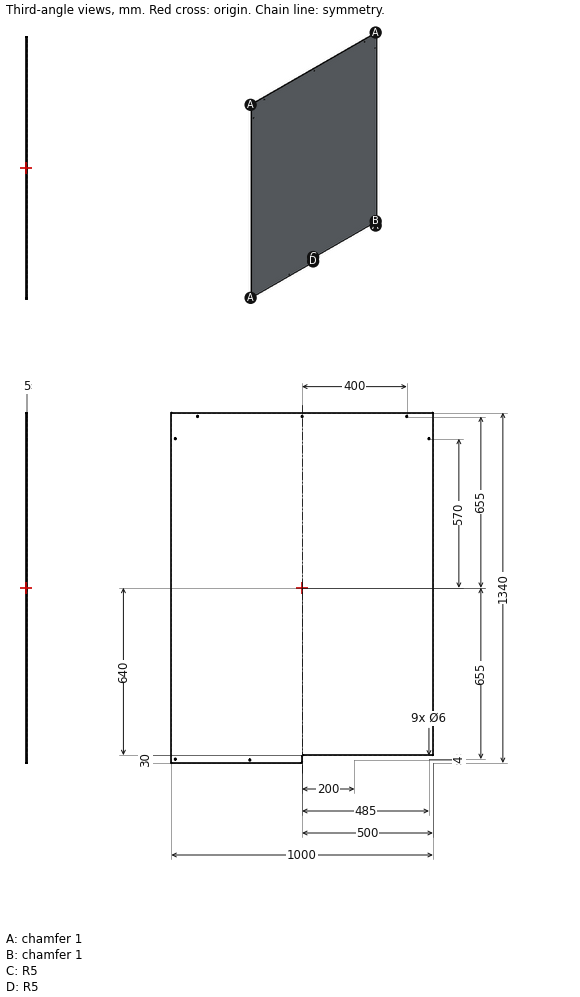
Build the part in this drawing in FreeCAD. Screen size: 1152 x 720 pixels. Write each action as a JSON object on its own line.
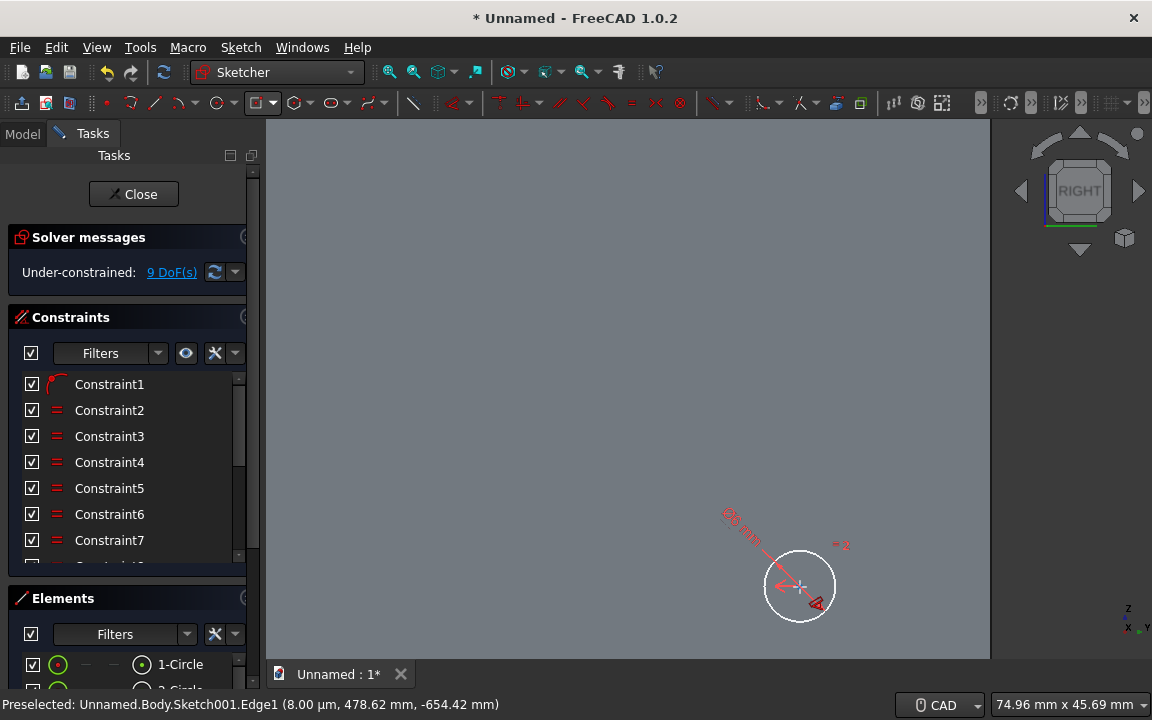
{"action": "left_click", "coordinate": [800, 586]}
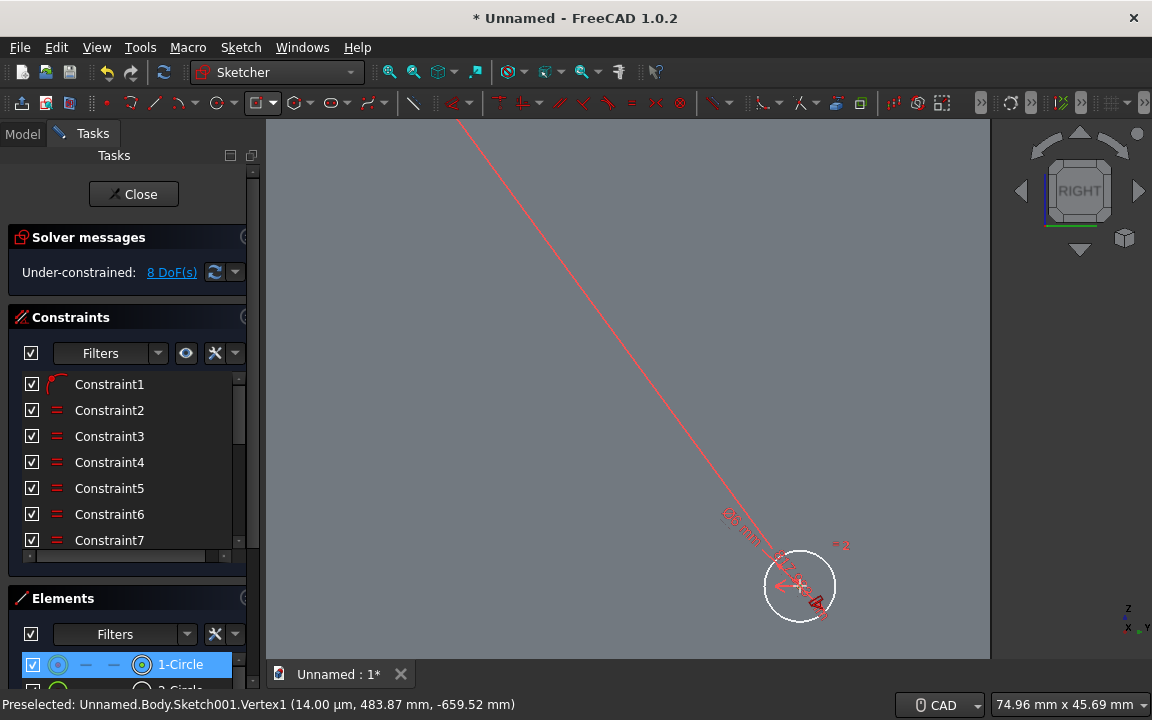
{"action": "scroll", "coordinate": [797, 602], "scroll_direction": "down", "scroll_amount": 18}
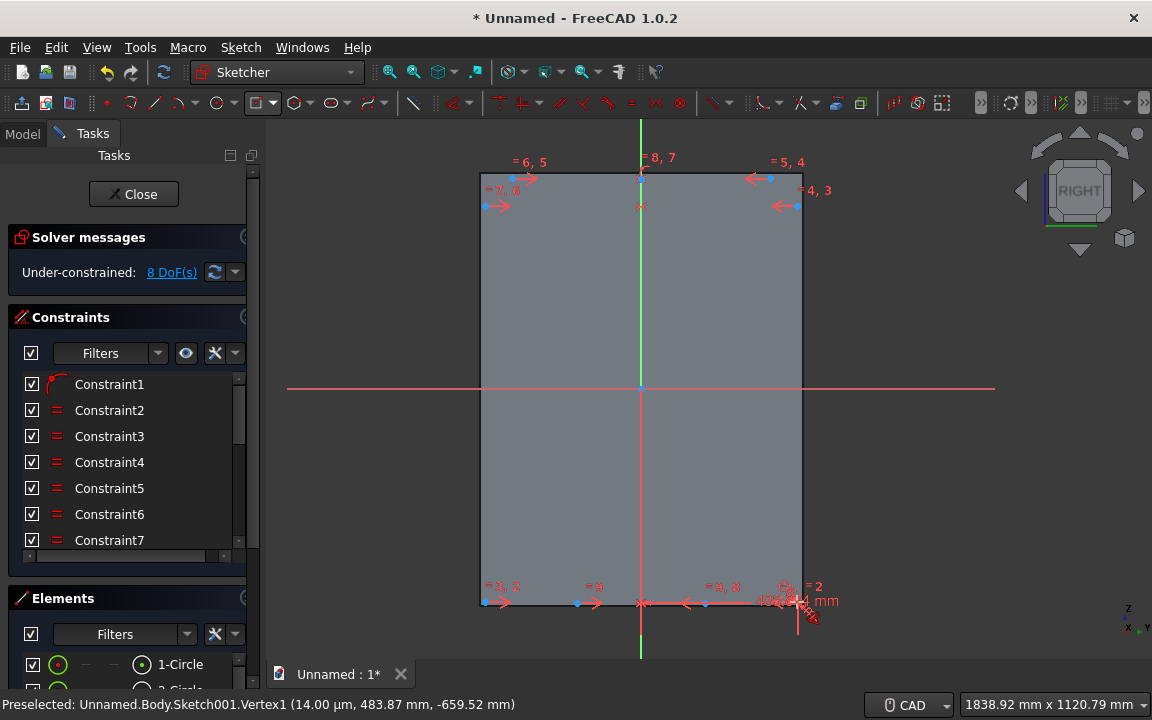
{"action": "scroll", "coordinate": [706, 603], "scroll_direction": "up", "scroll_amount": 18}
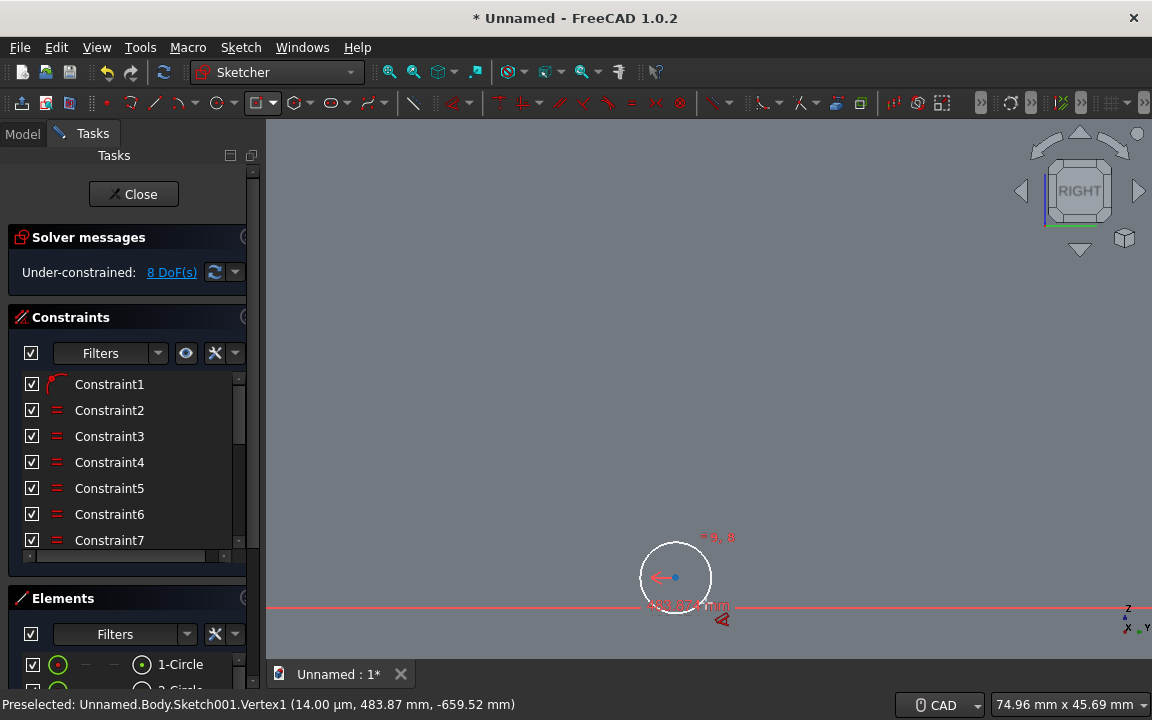
{"action": "left_click", "coordinate": [676, 578]}
{"action": "left_click", "coordinate": [618, 564]}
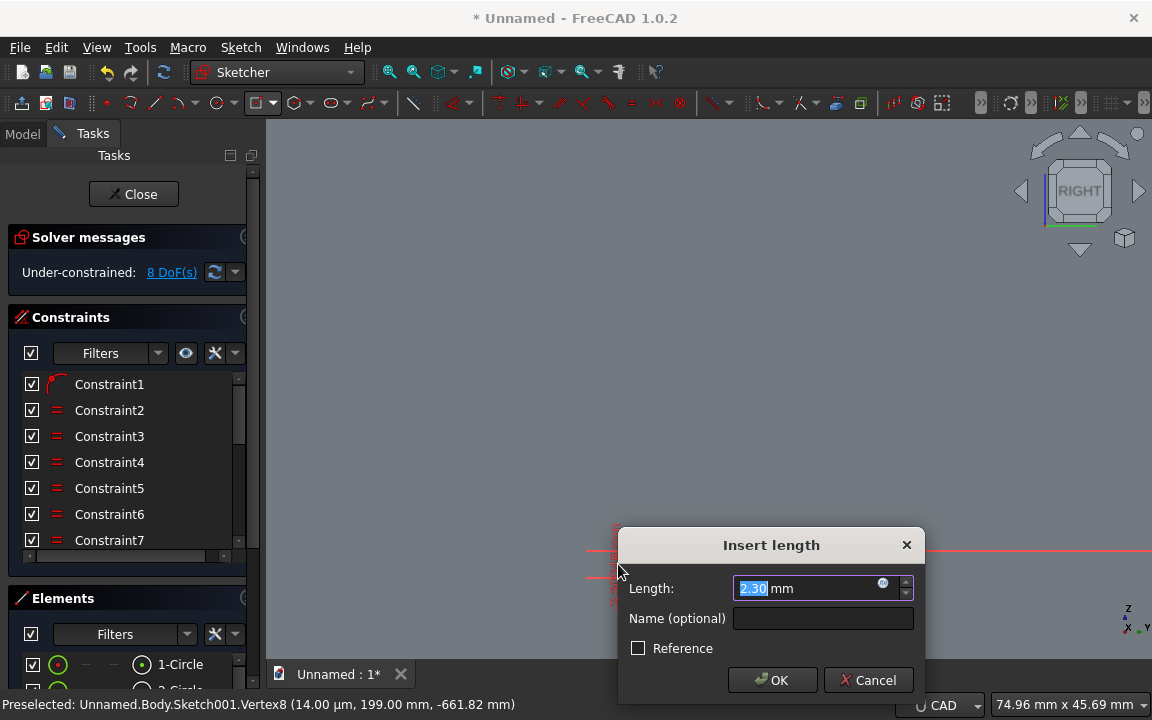
{"action": "type", "text": "4"}
{"action": "key", "text": "Return"}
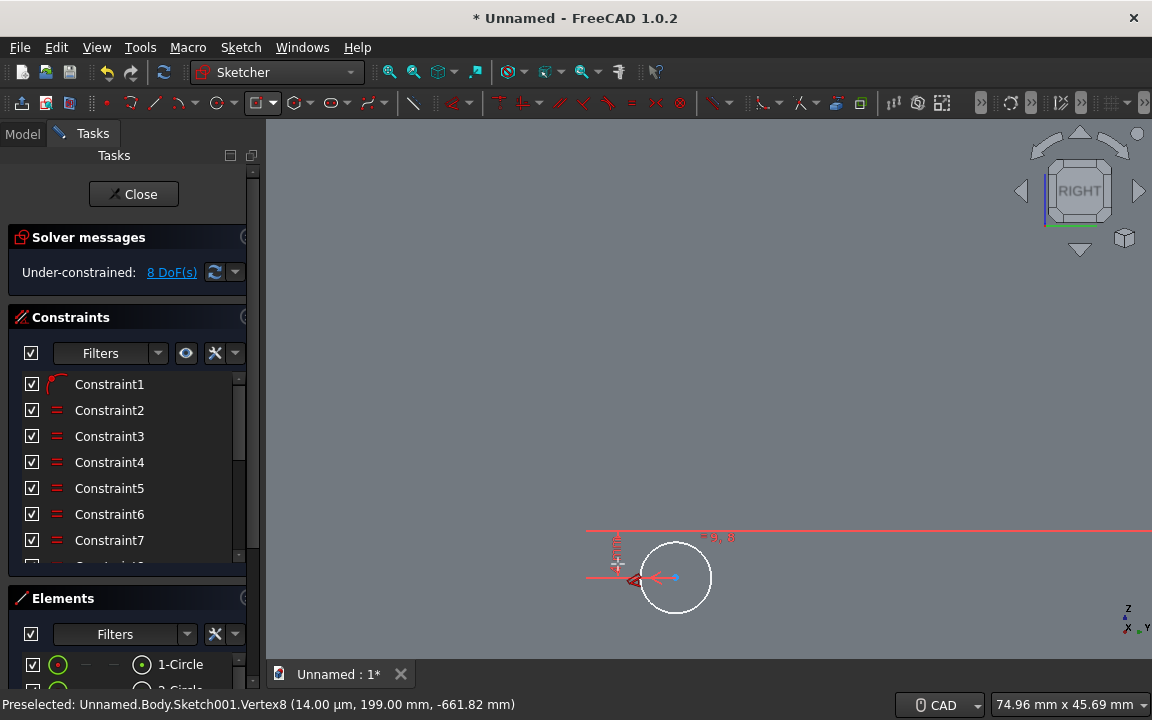
{"action": "scroll", "coordinate": [706, 603], "scroll_direction": "down", "scroll_amount": 18}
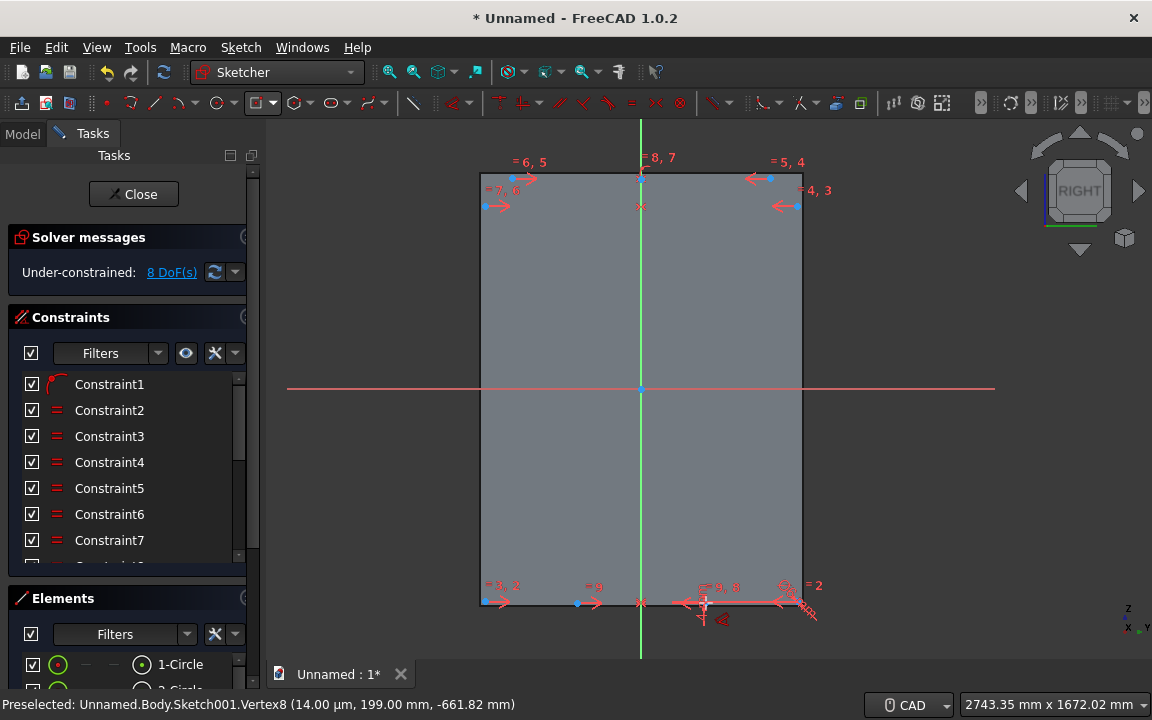
{"action": "left_click", "coordinate": [798, 602]}
{"action": "left_click", "coordinate": [720, 355]}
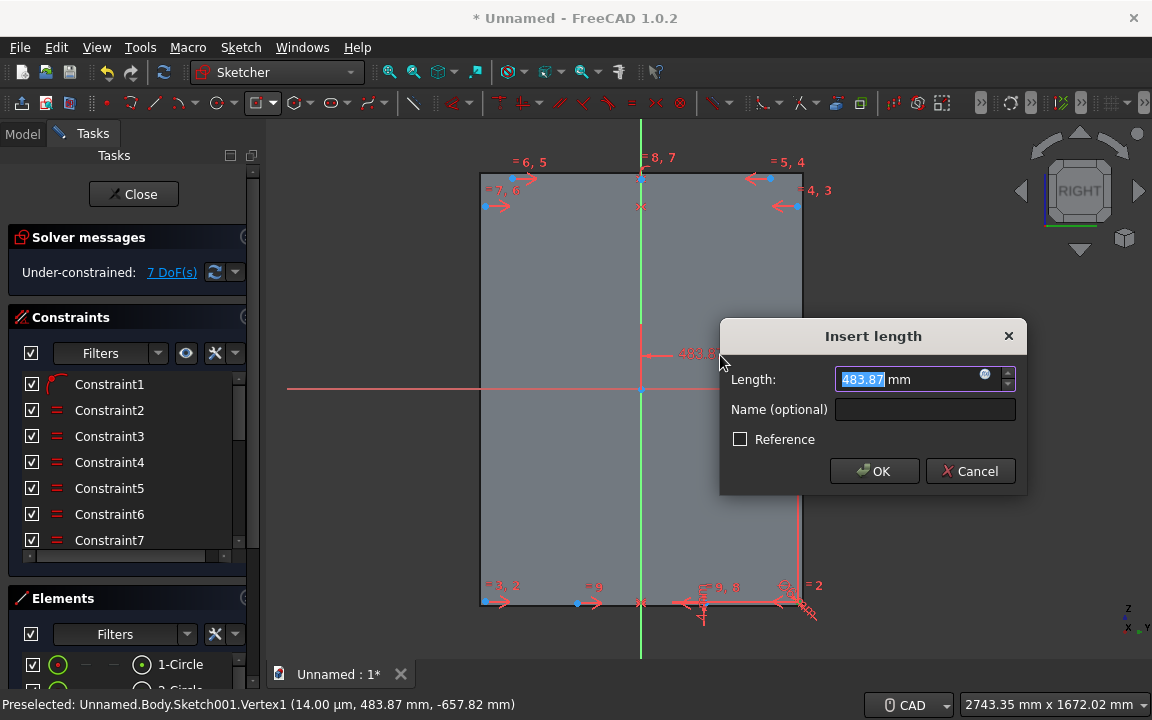
{"action": "type", "text": "485"}
{"action": "key", "text": "Return"}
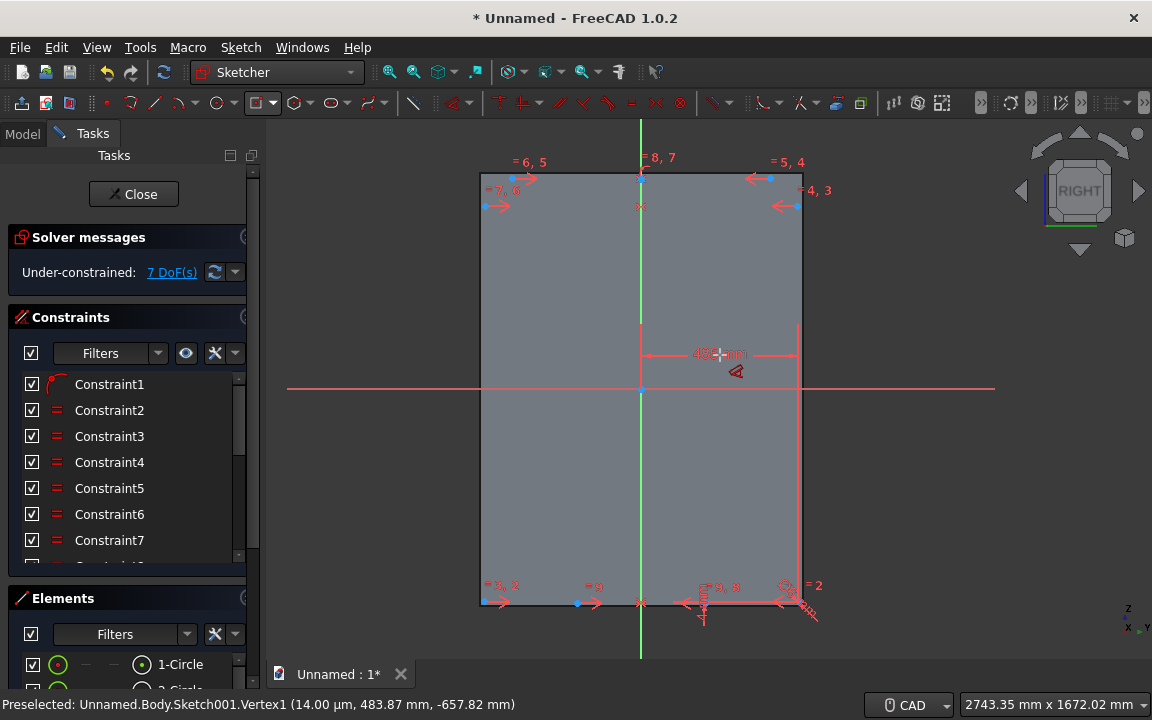
{"action": "left_click", "coordinate": [798, 602]}
{"action": "left_click", "coordinate": [832, 496]}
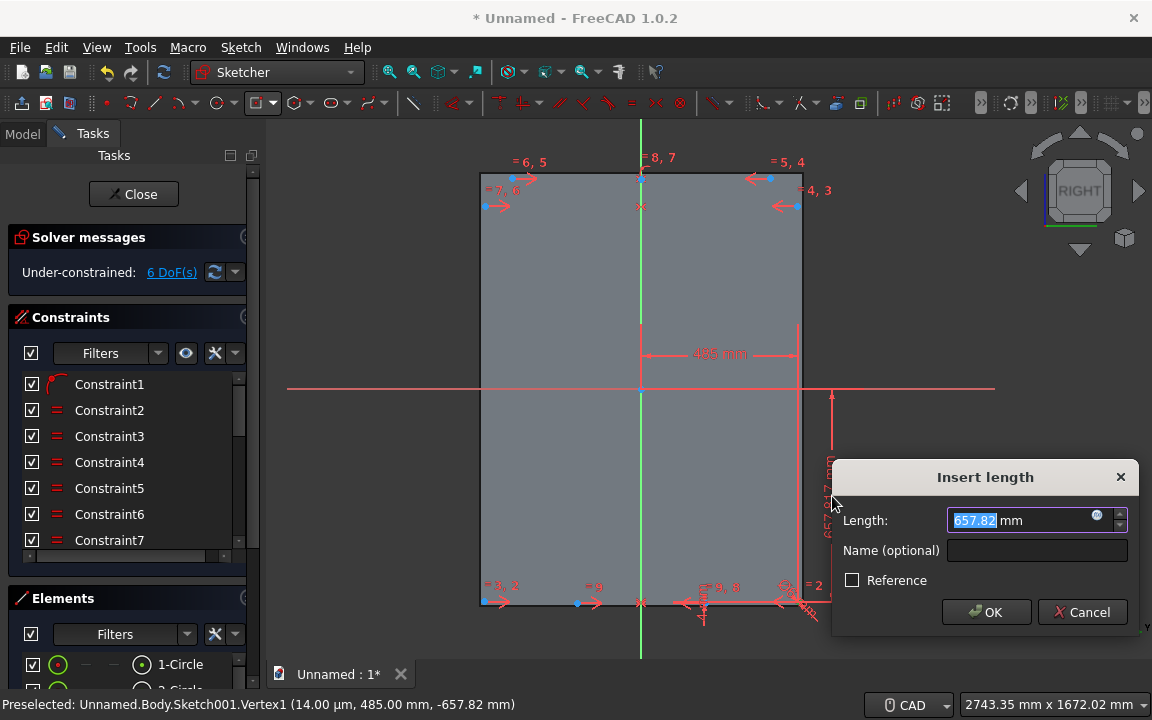
{"action": "type", "text": "655"}
{"action": "key", "text": "Return"}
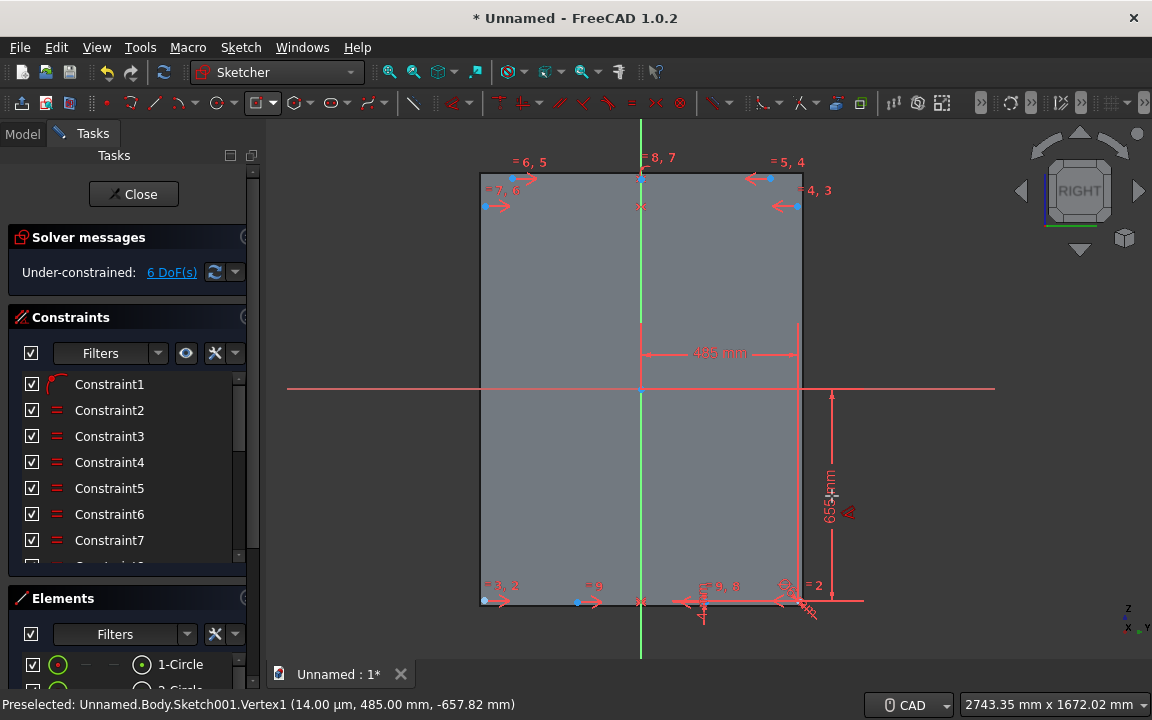
{"action": "left_click", "coordinate": [798, 206]}
{"action": "left_click", "coordinate": [720, 172]}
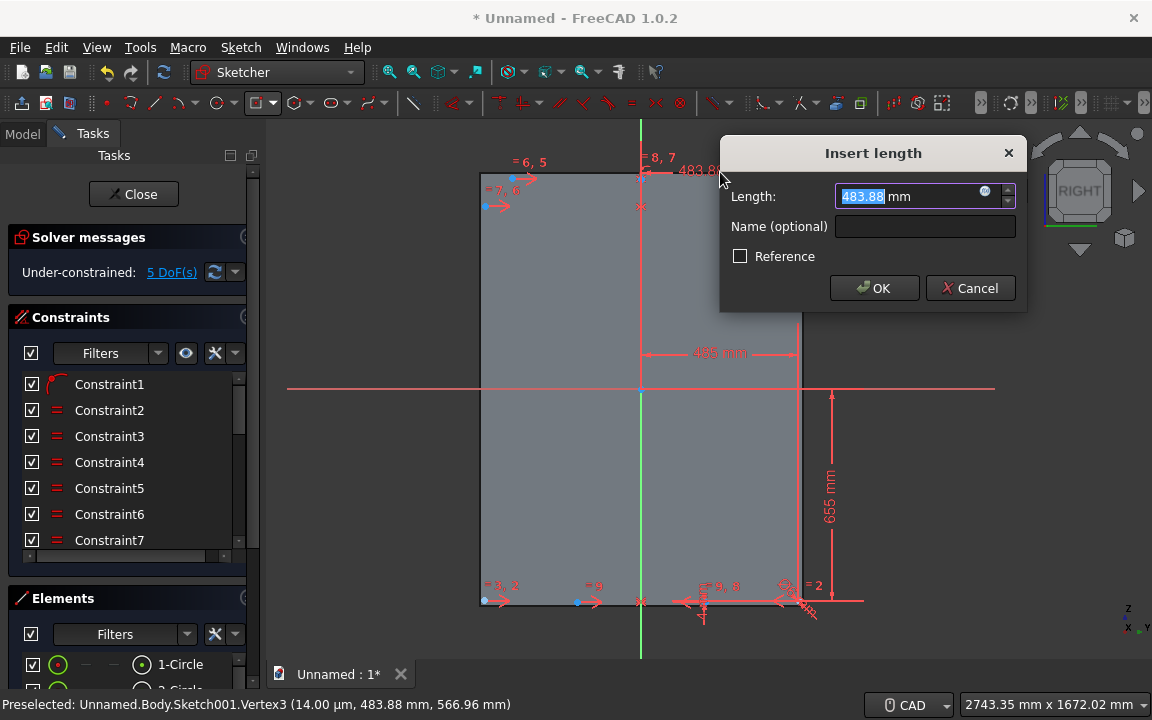
{"action": "type", "text": "485"}
{"action": "key", "text": "Return"}